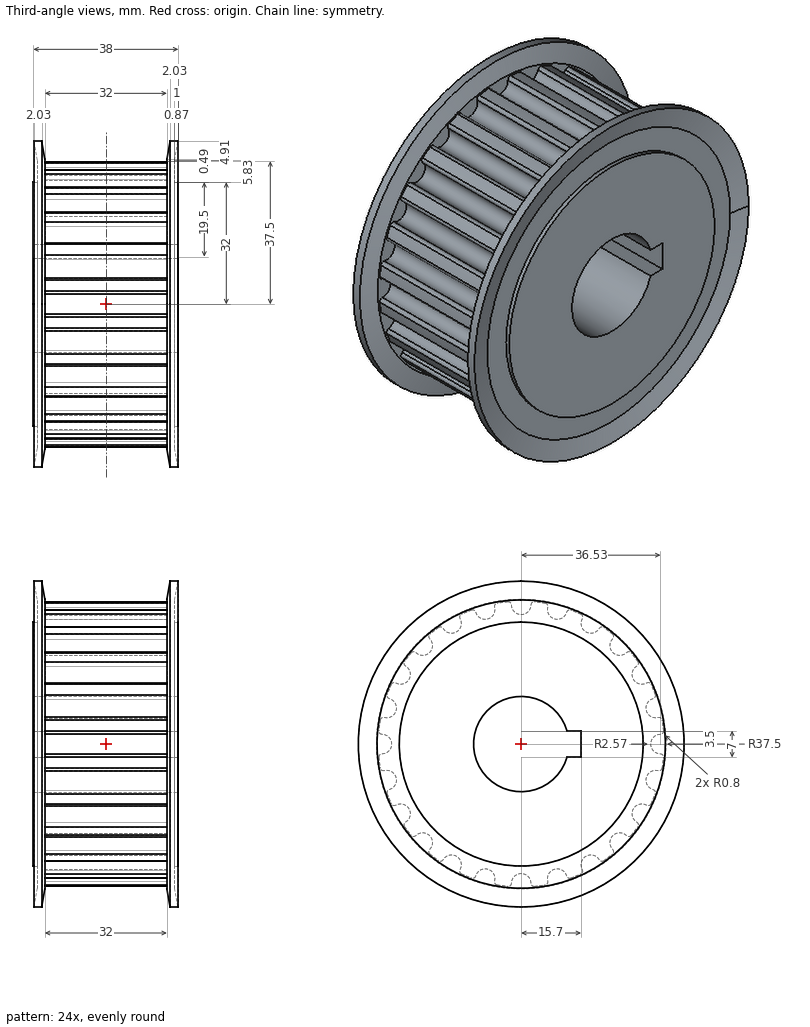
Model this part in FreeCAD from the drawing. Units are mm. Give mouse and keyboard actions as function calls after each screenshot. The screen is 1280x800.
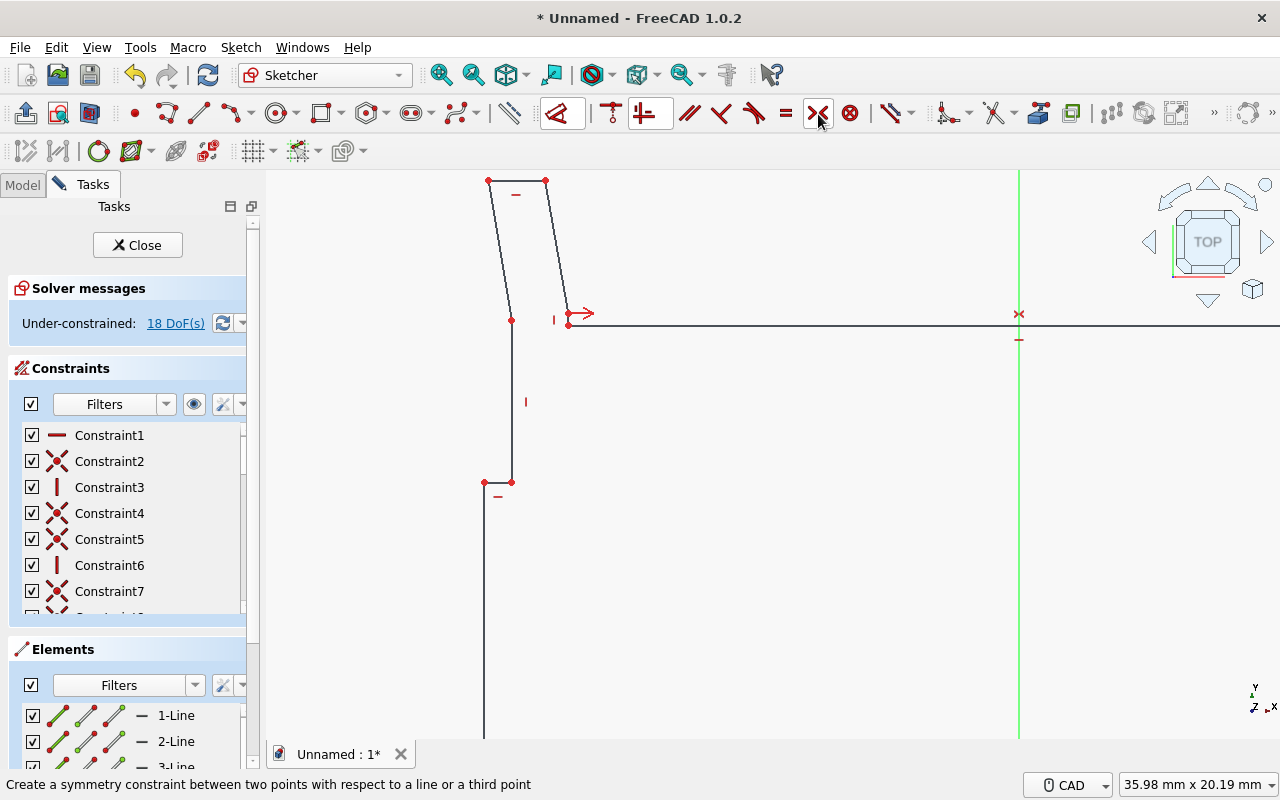
scroll(569, 314, down, 6)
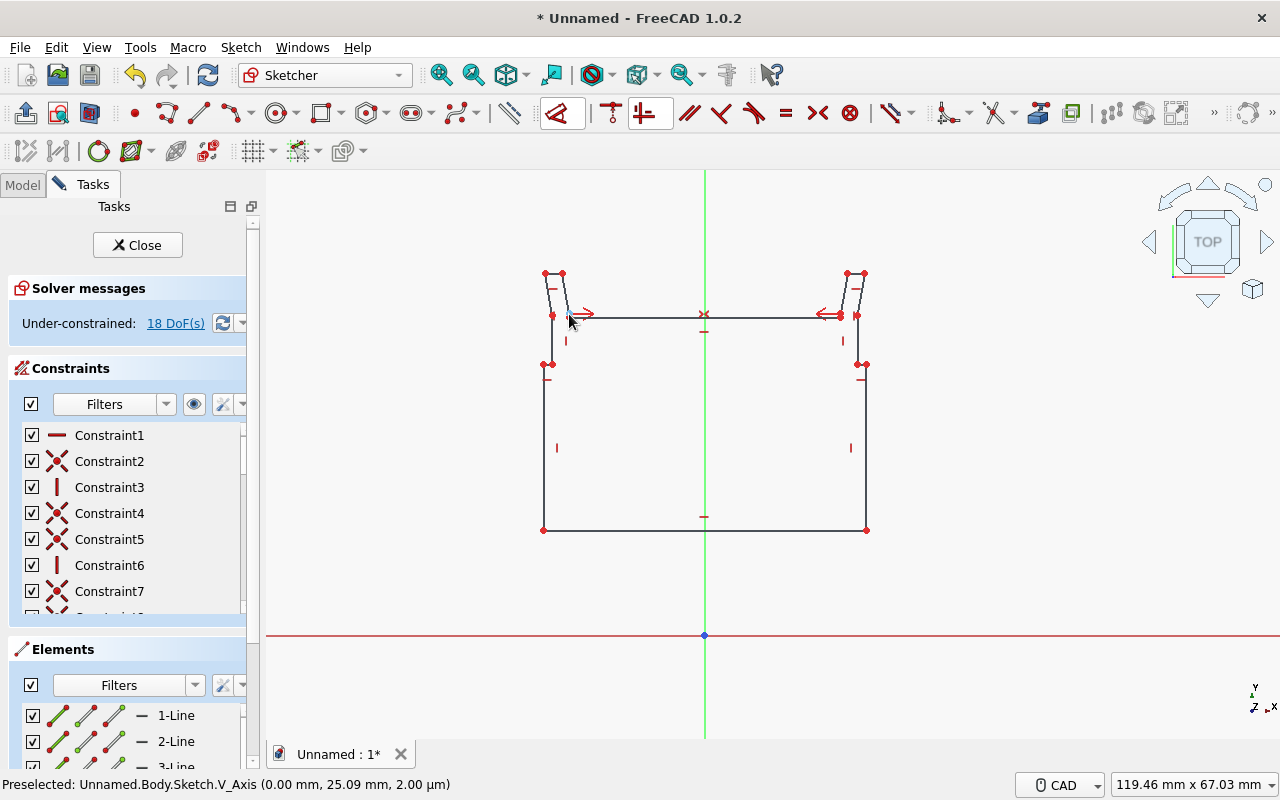
click(848, 274)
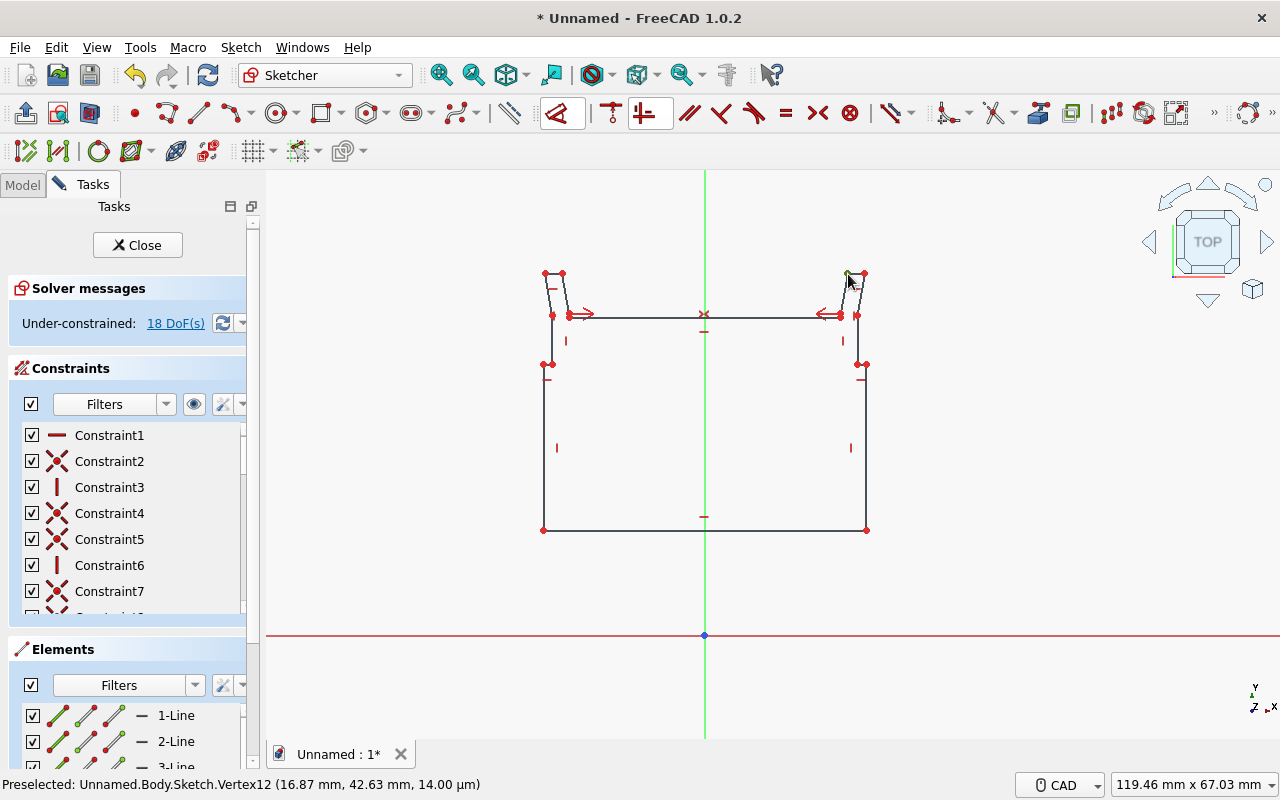
click(562, 274)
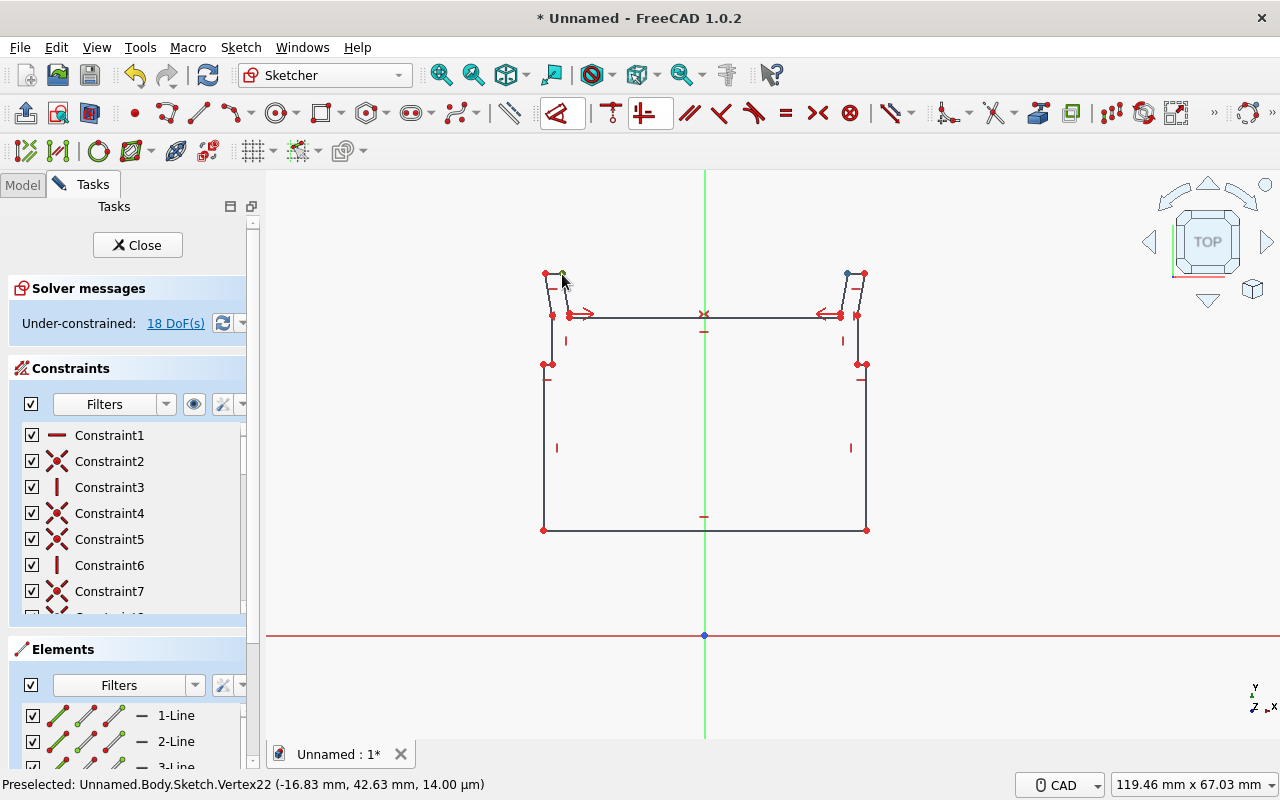
click(705, 674)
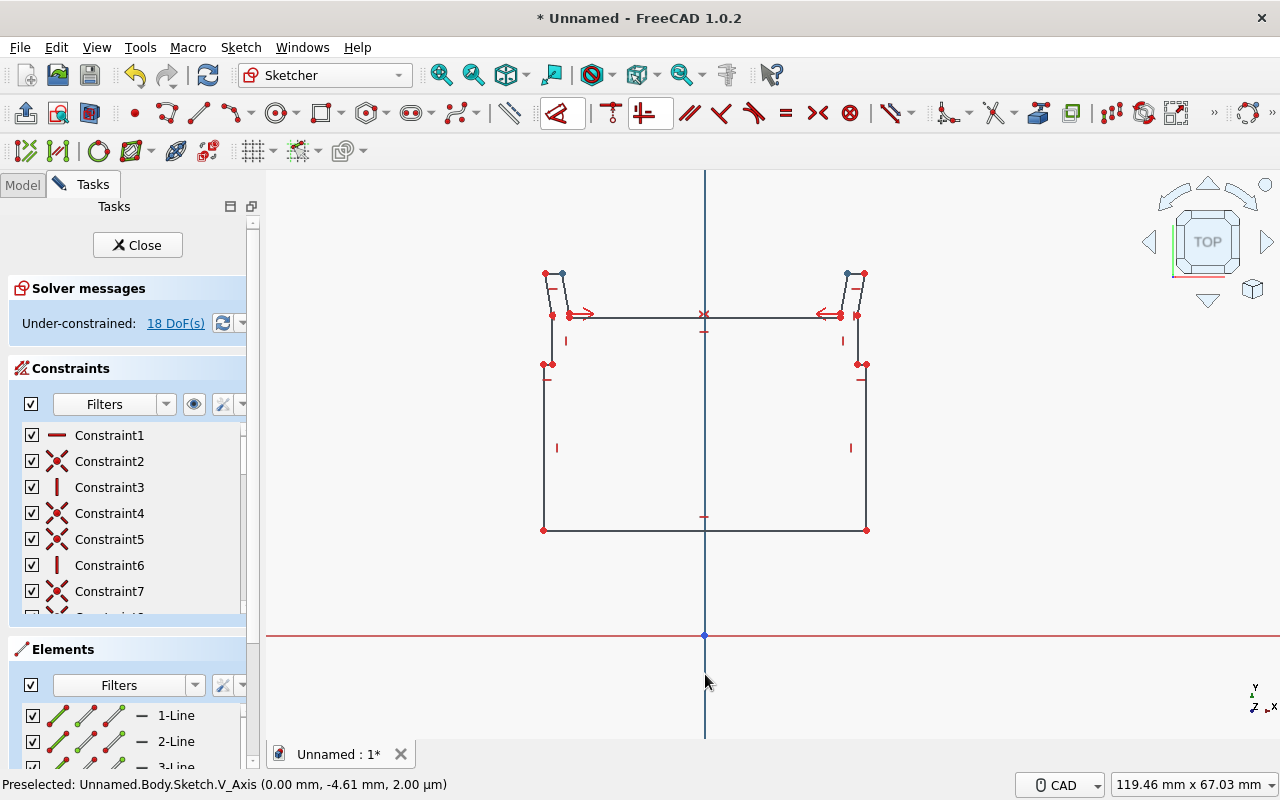
click(818, 114)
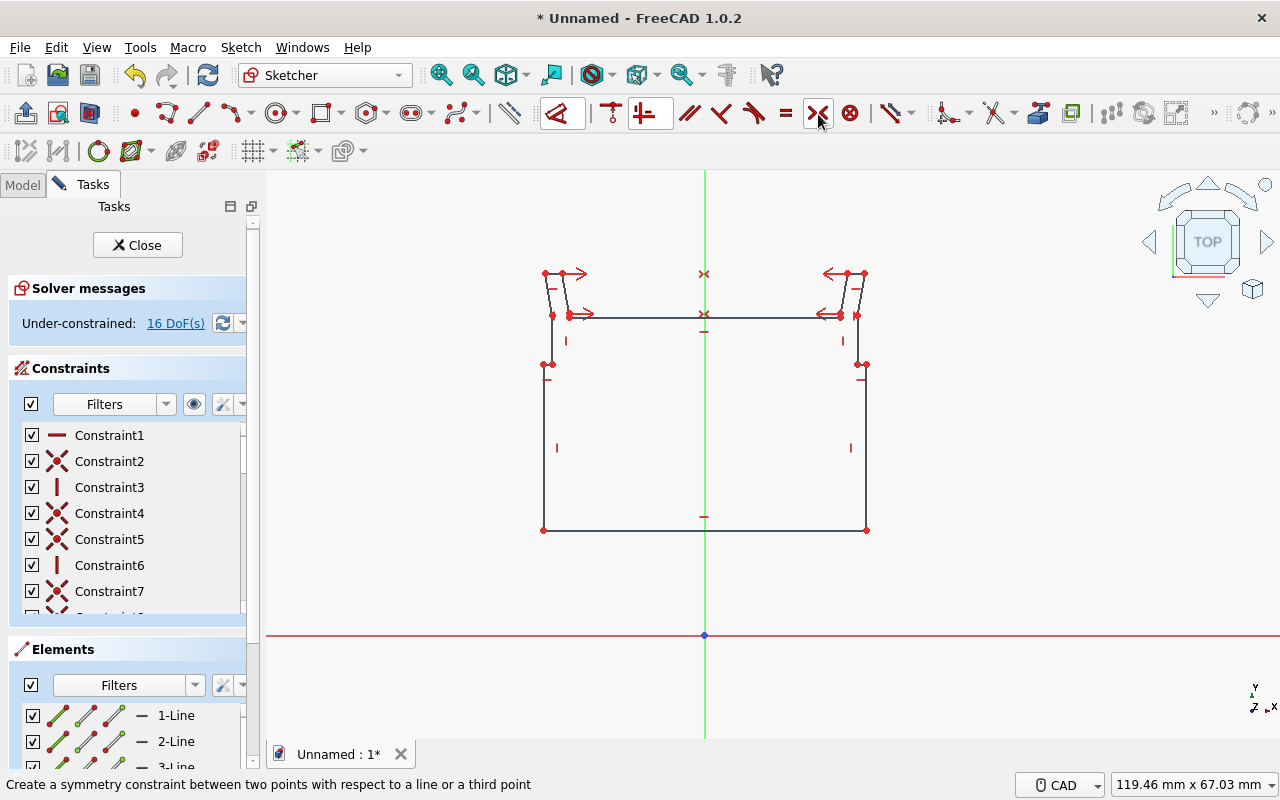
click(858, 315)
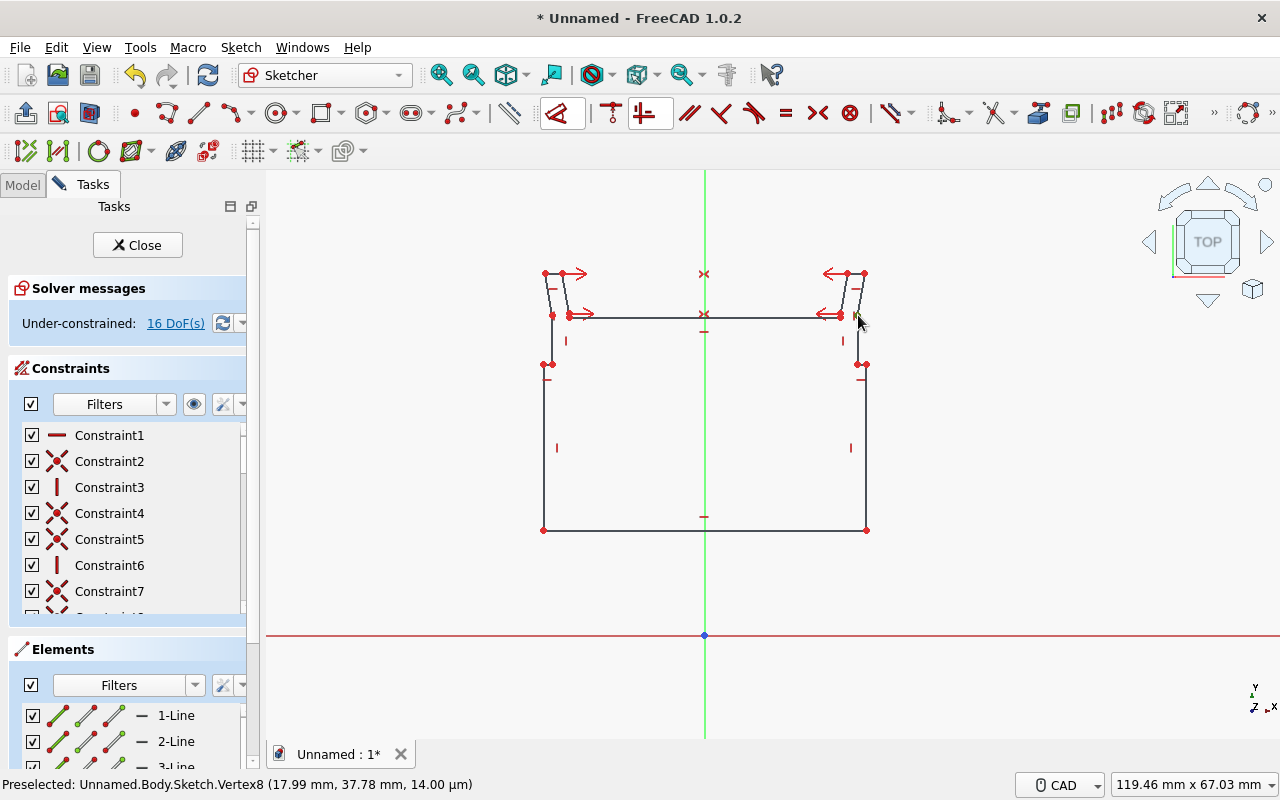
click(552, 316)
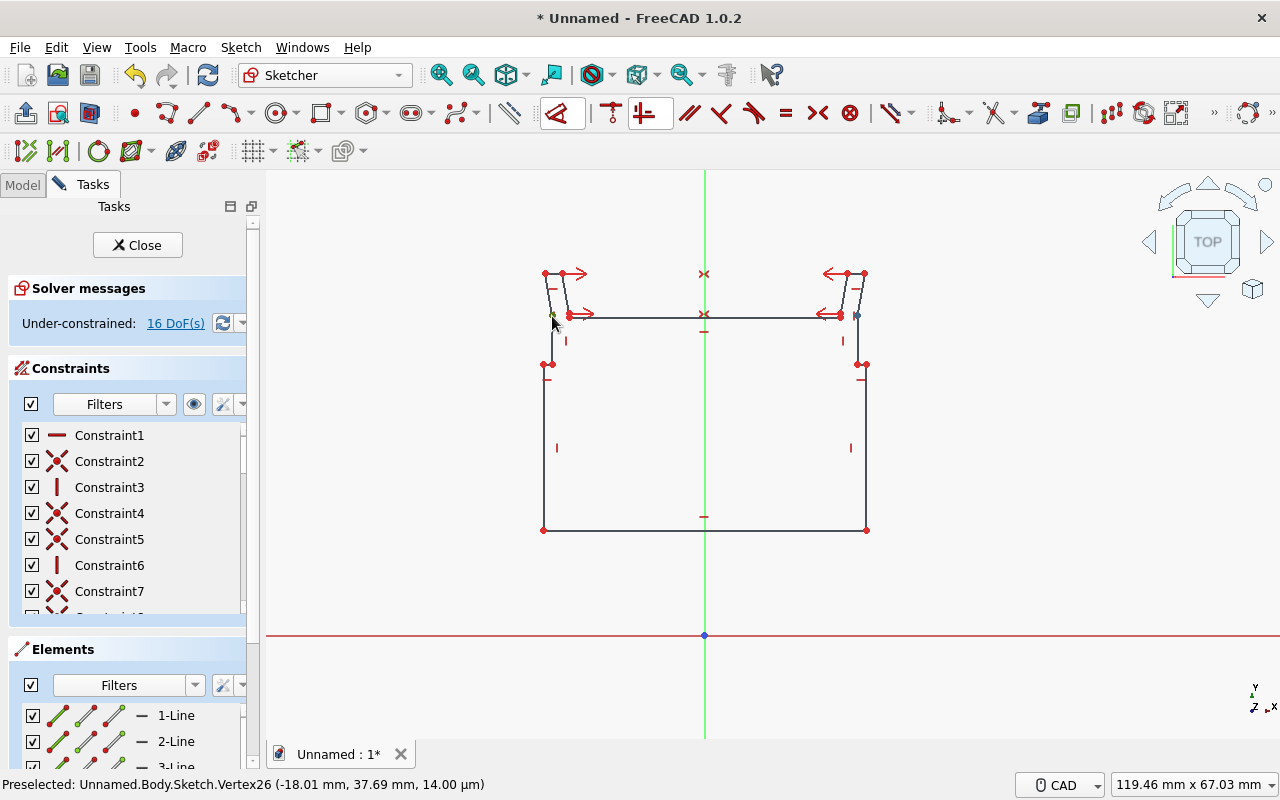
click(705, 674)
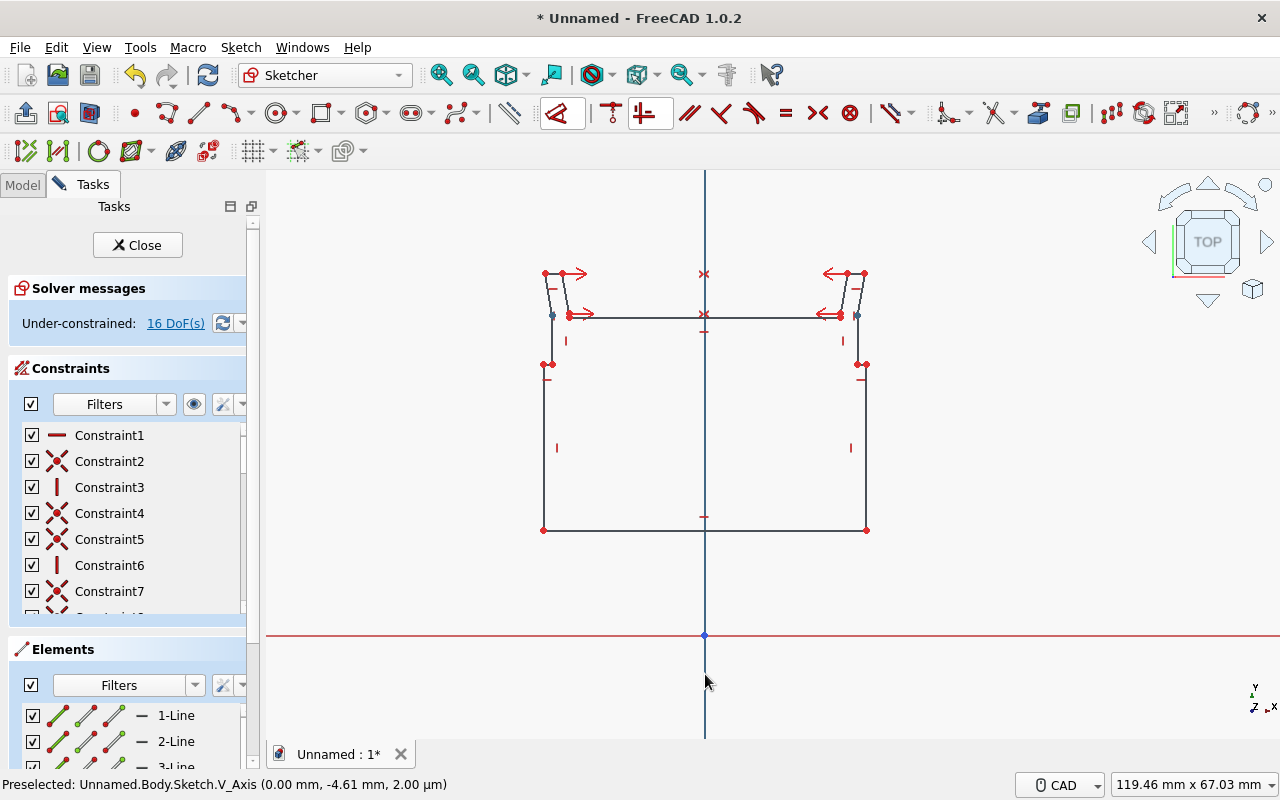
click(818, 114)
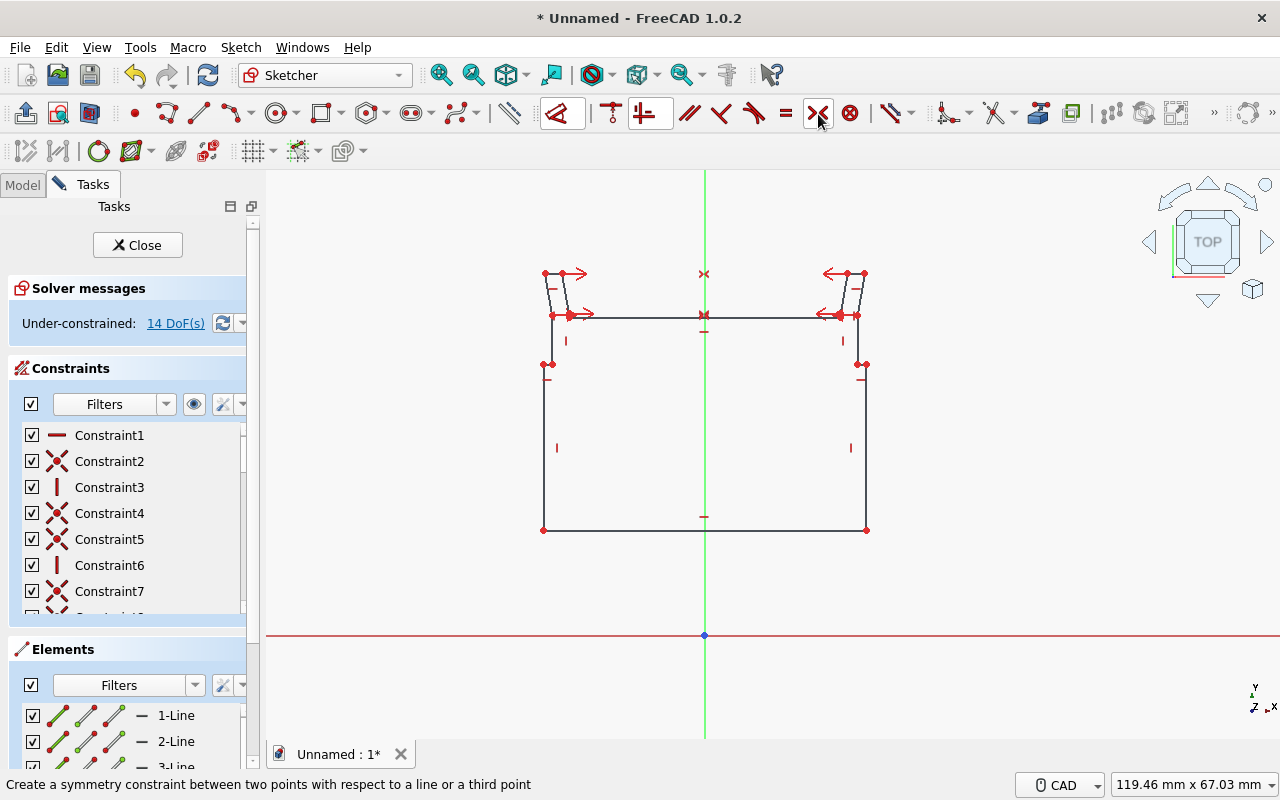
scroll(866, 365, up, 2)